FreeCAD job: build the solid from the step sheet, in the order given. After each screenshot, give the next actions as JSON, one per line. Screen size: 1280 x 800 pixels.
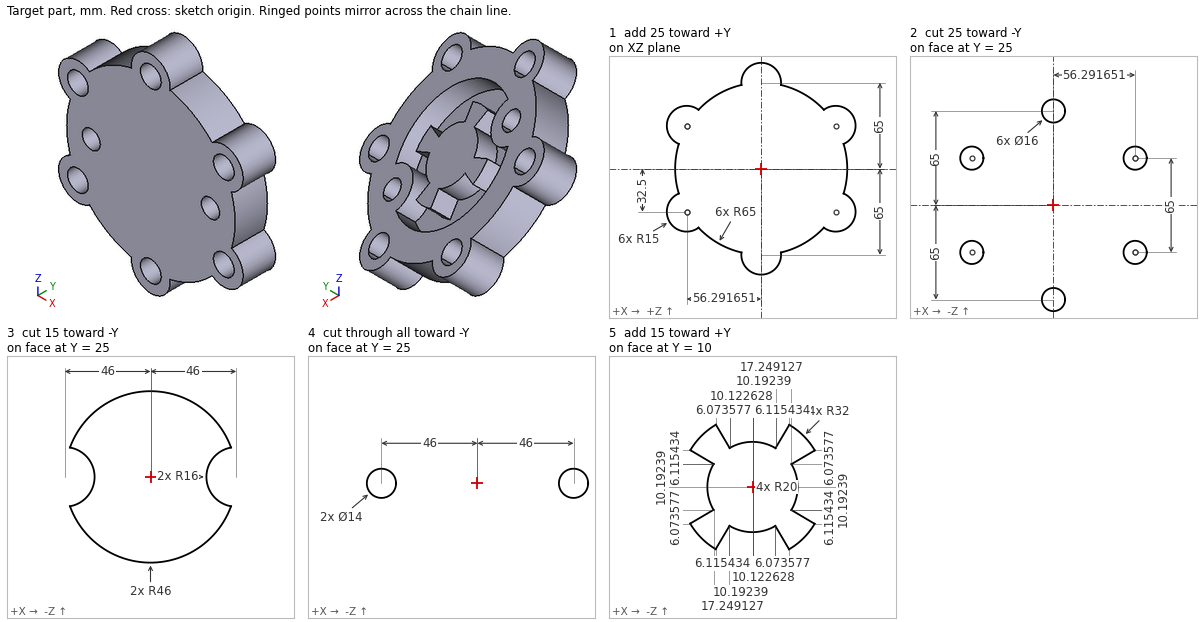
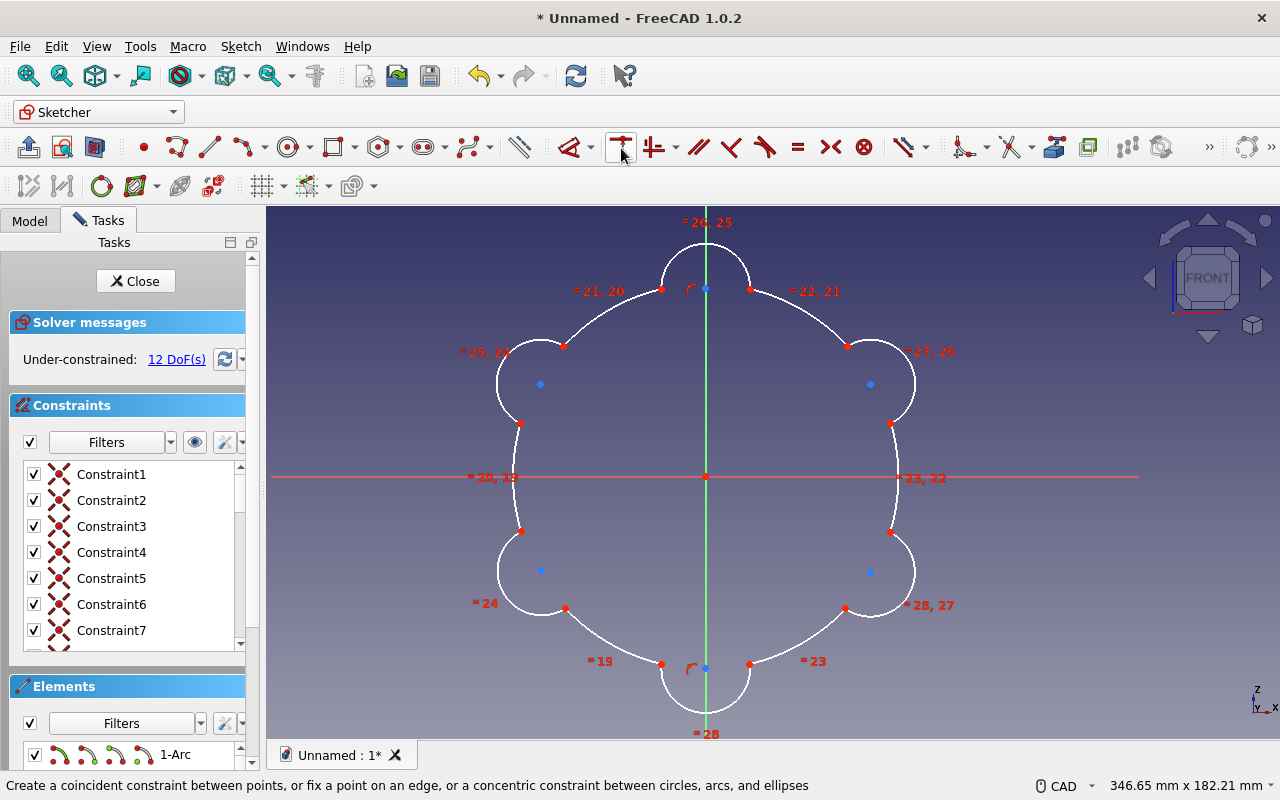
{"action": "left_click", "coordinate": [542, 571]}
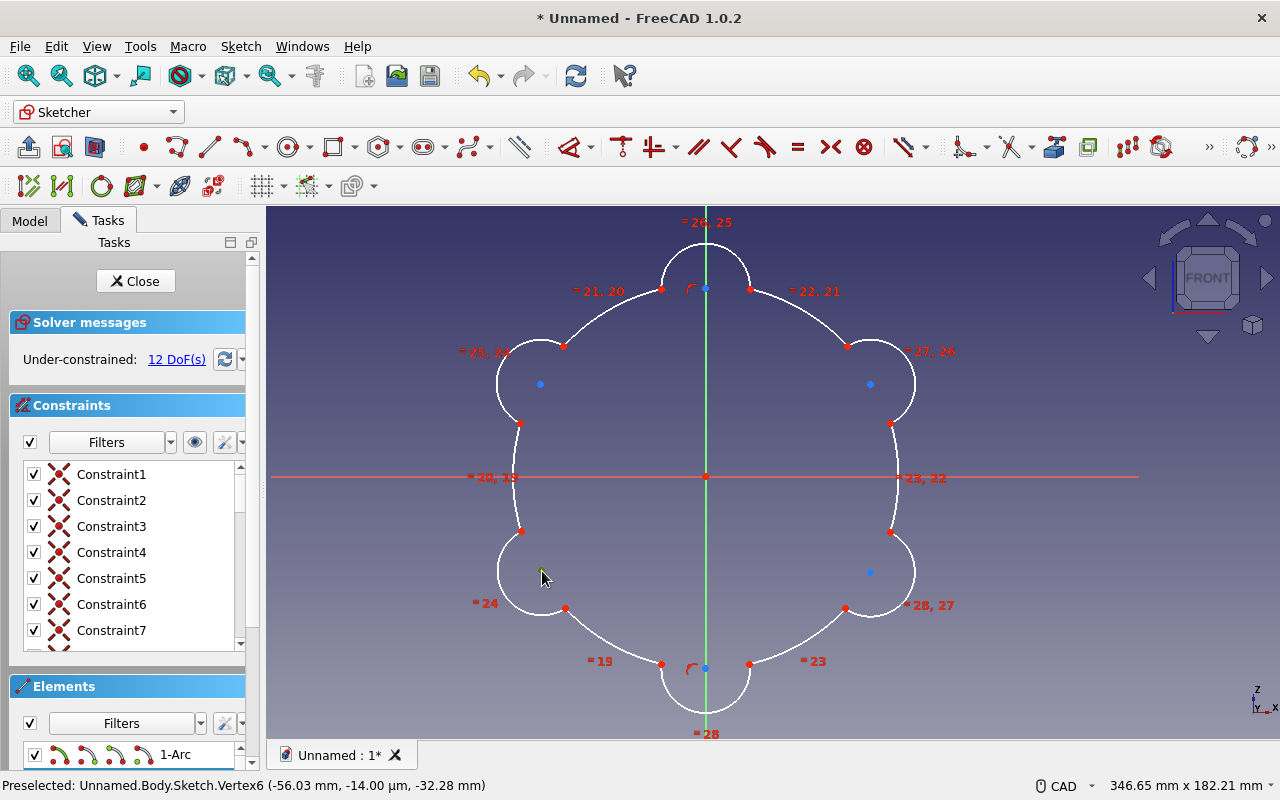
{"action": "left_click", "coordinate": [541, 384]}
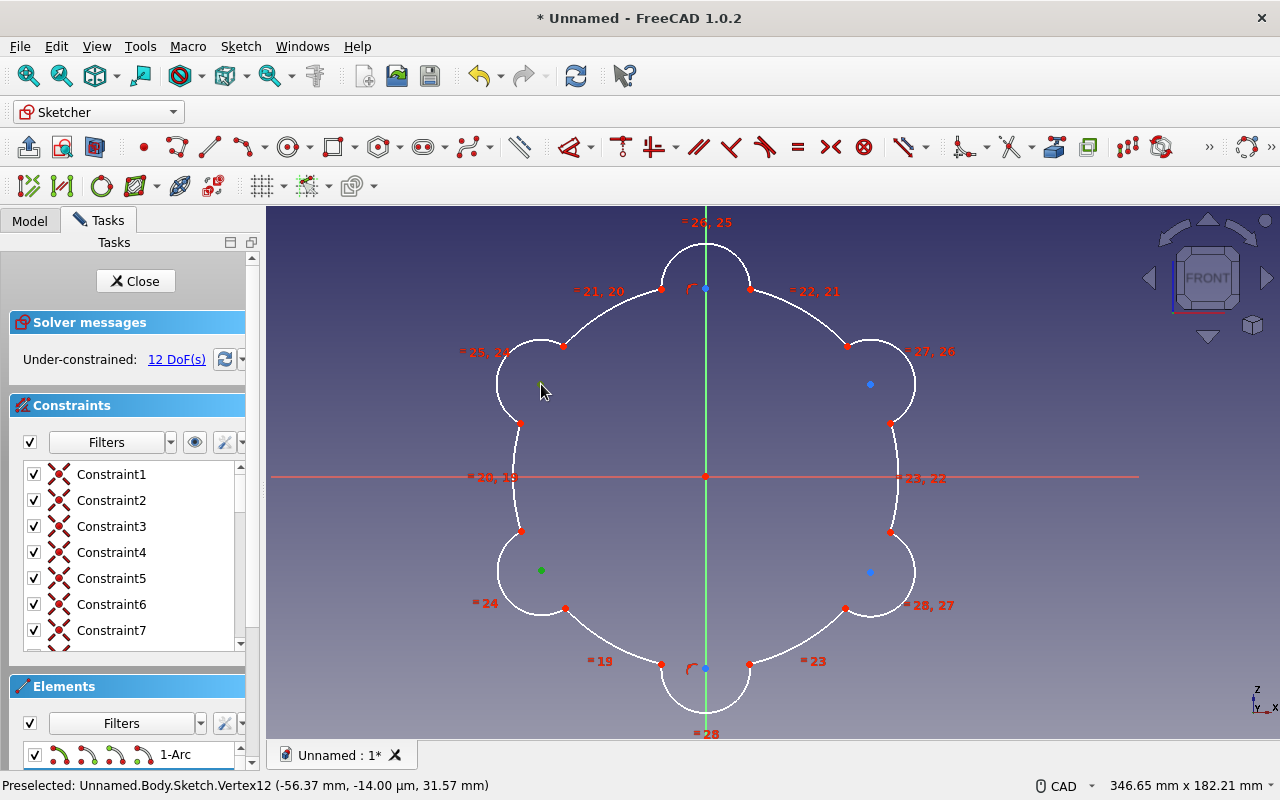
{"action": "left_click", "coordinate": [353, 477]}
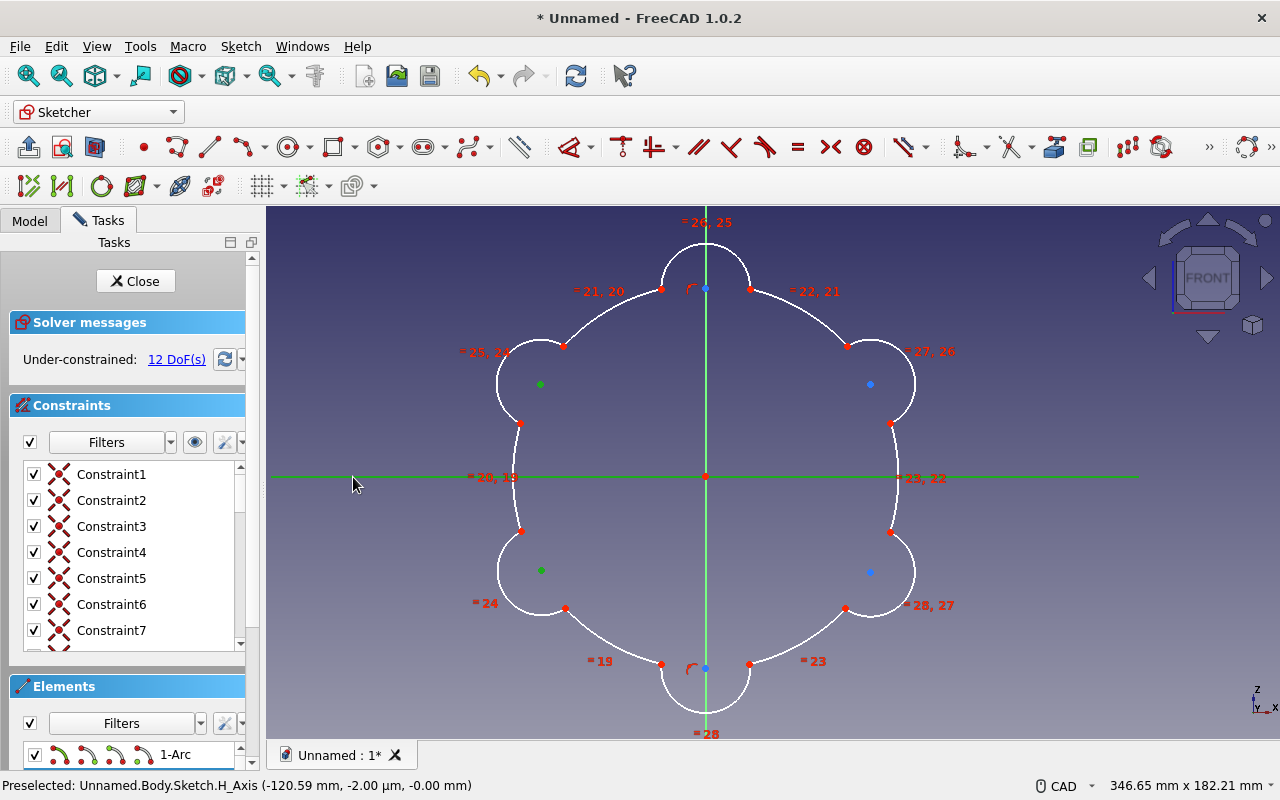
{"action": "left_click", "coordinate": [831, 148]}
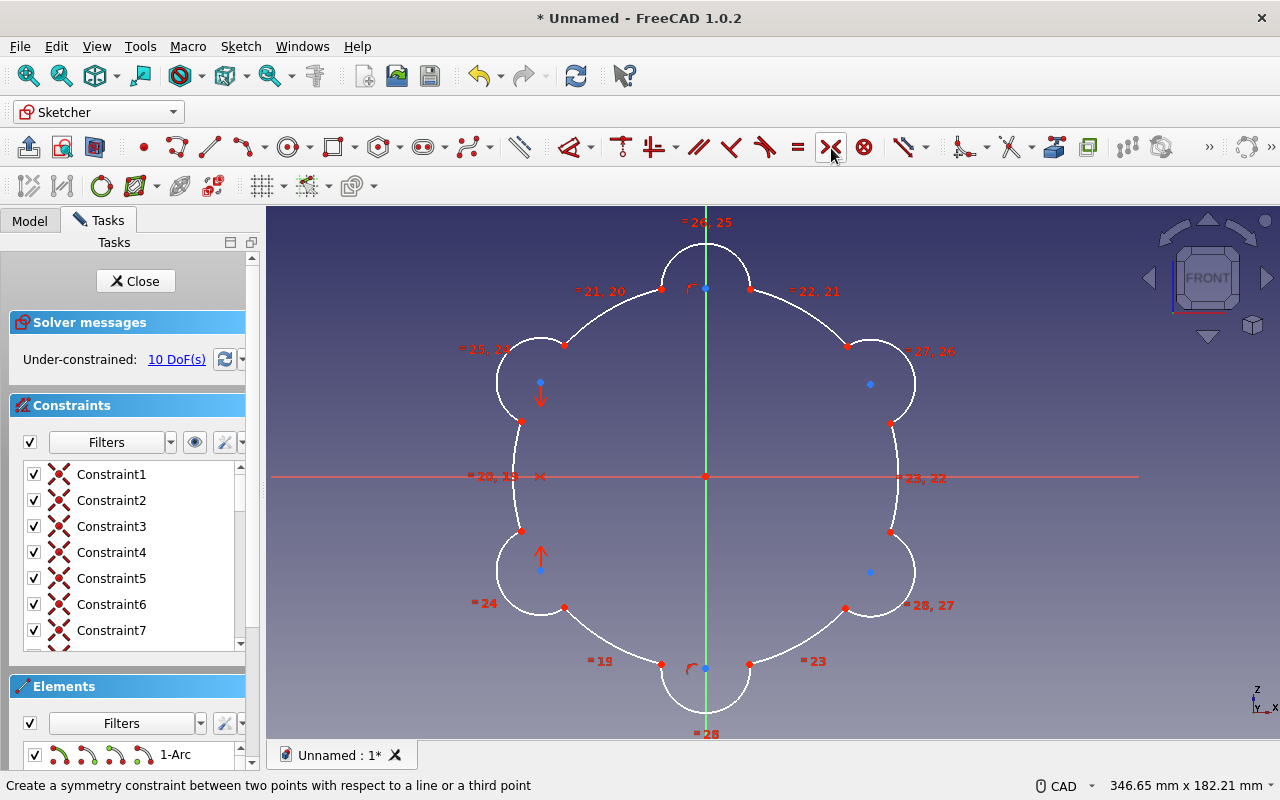
{"action": "left_click", "coordinate": [541, 382]}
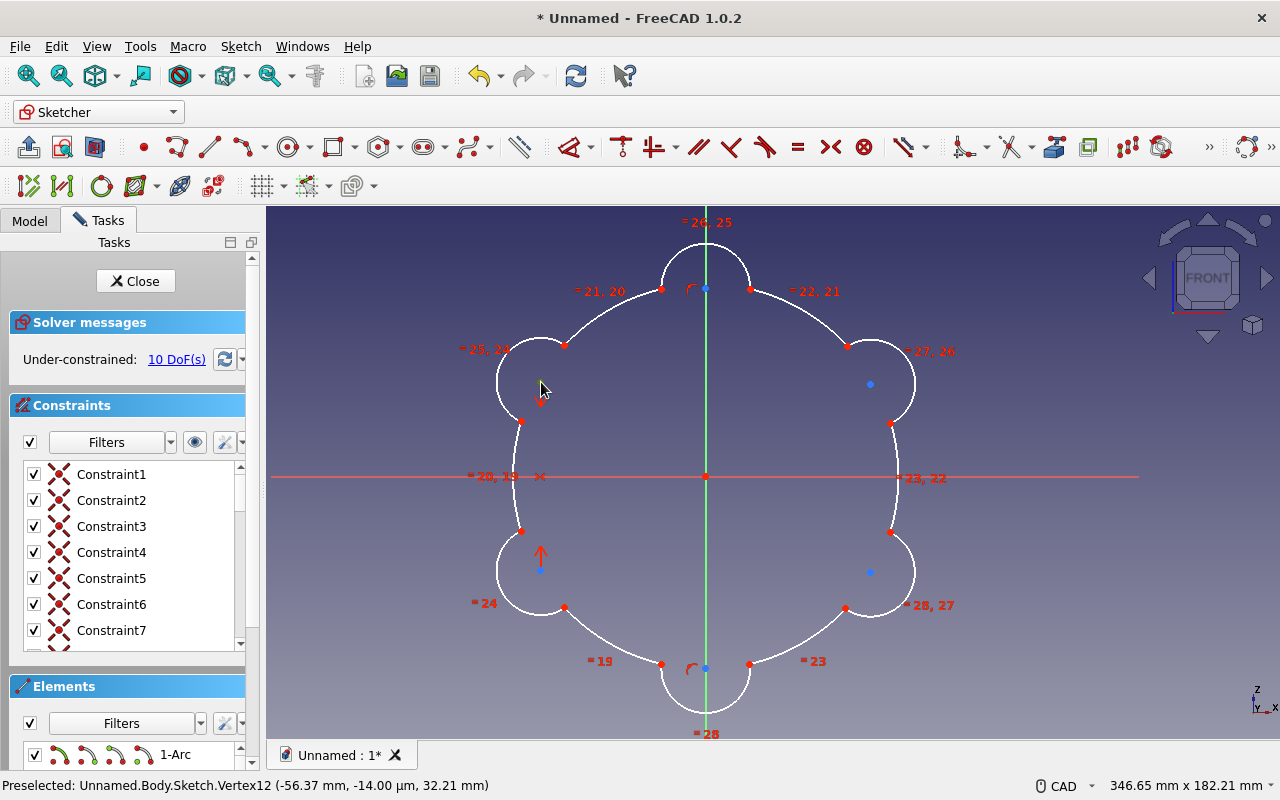
{"action": "left_click", "coordinate": [871, 384]}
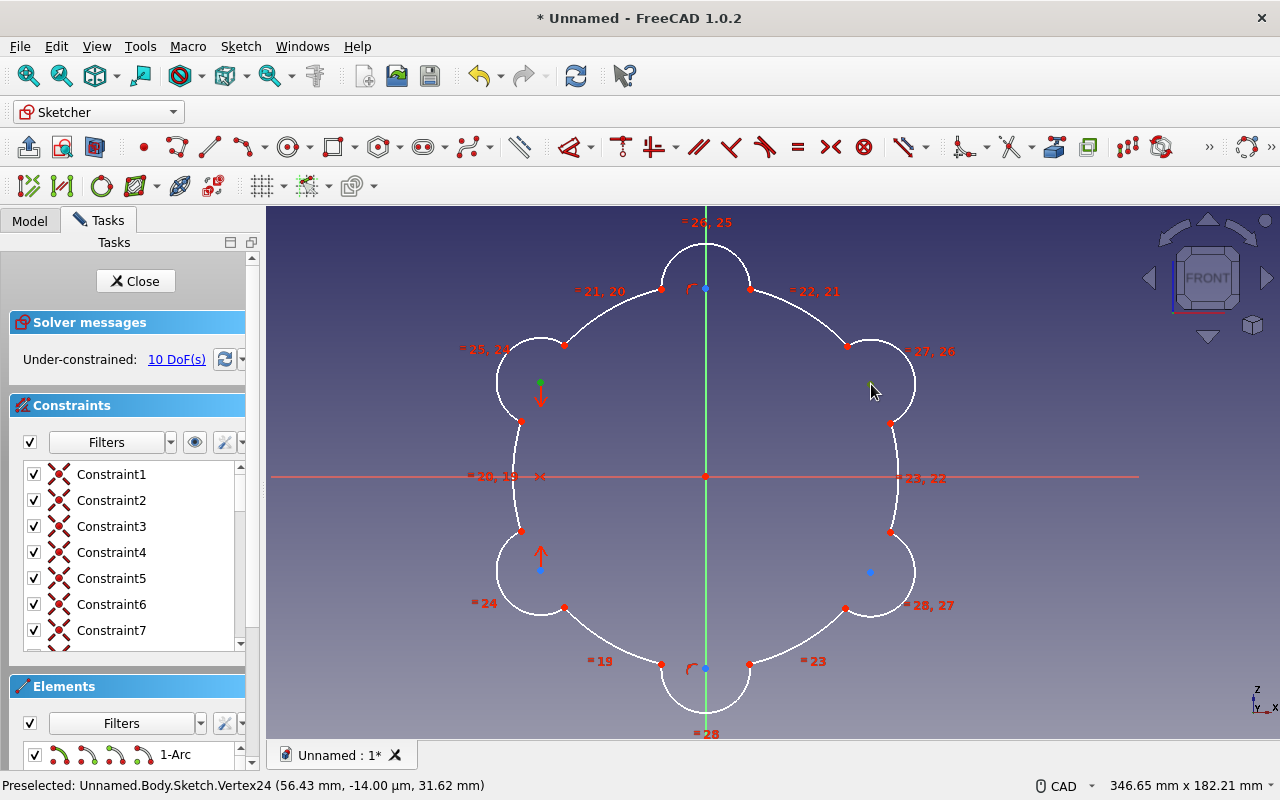
{"action": "left_click", "coordinate": [706, 677]}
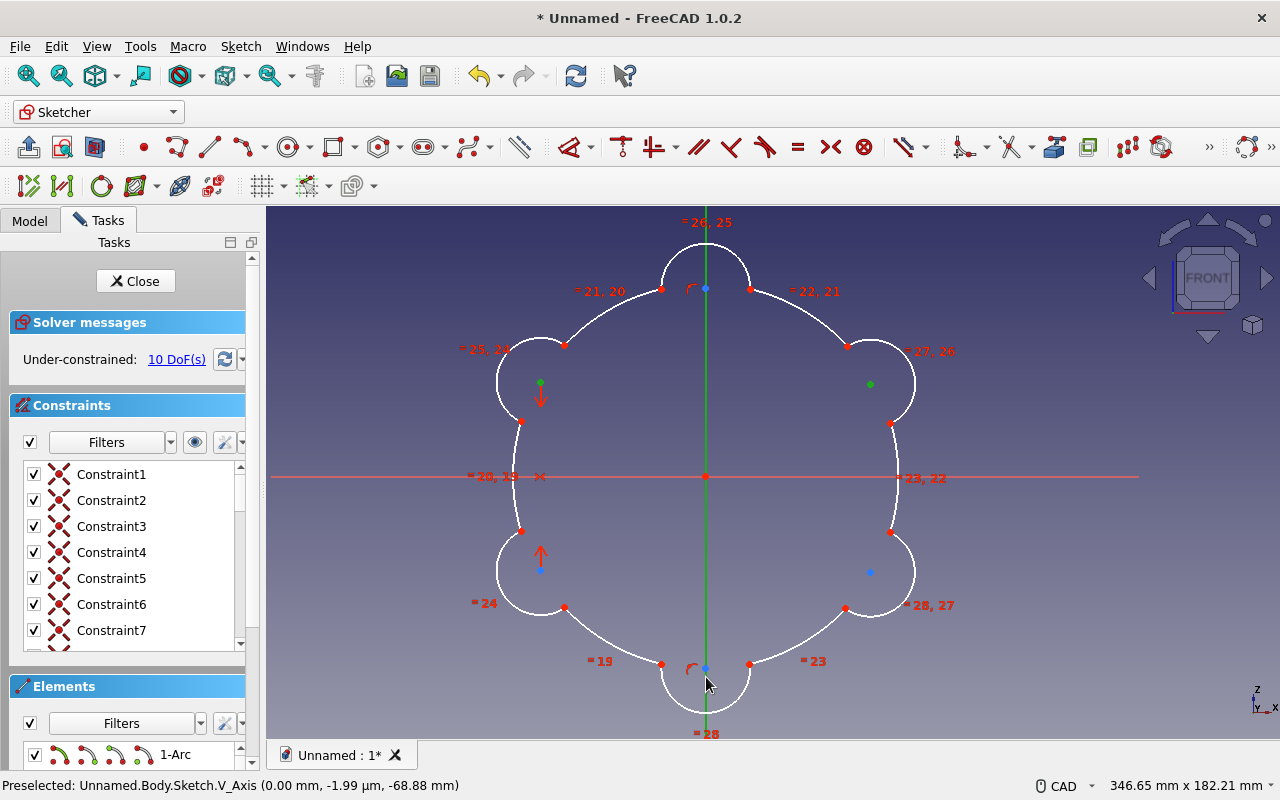
{"action": "left_click", "coordinate": [831, 148]}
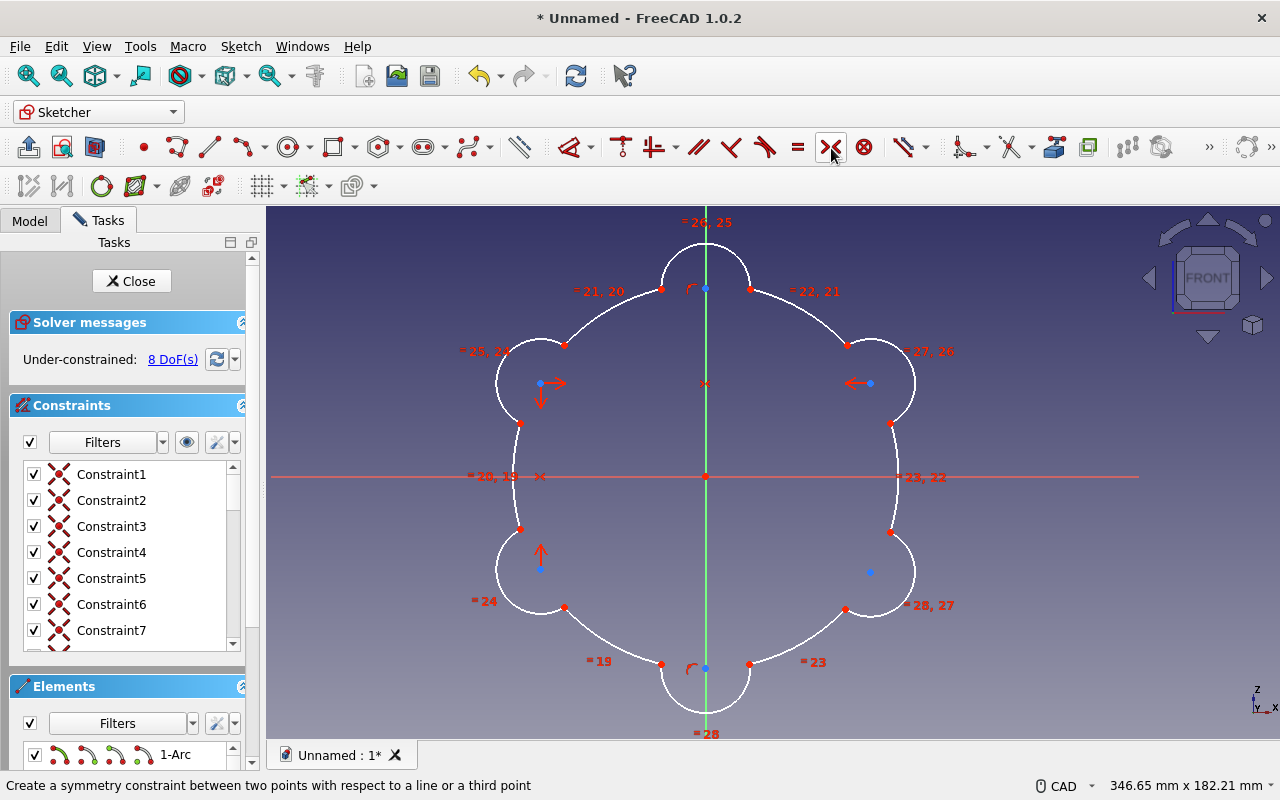
{"action": "left_click", "coordinate": [541, 570]}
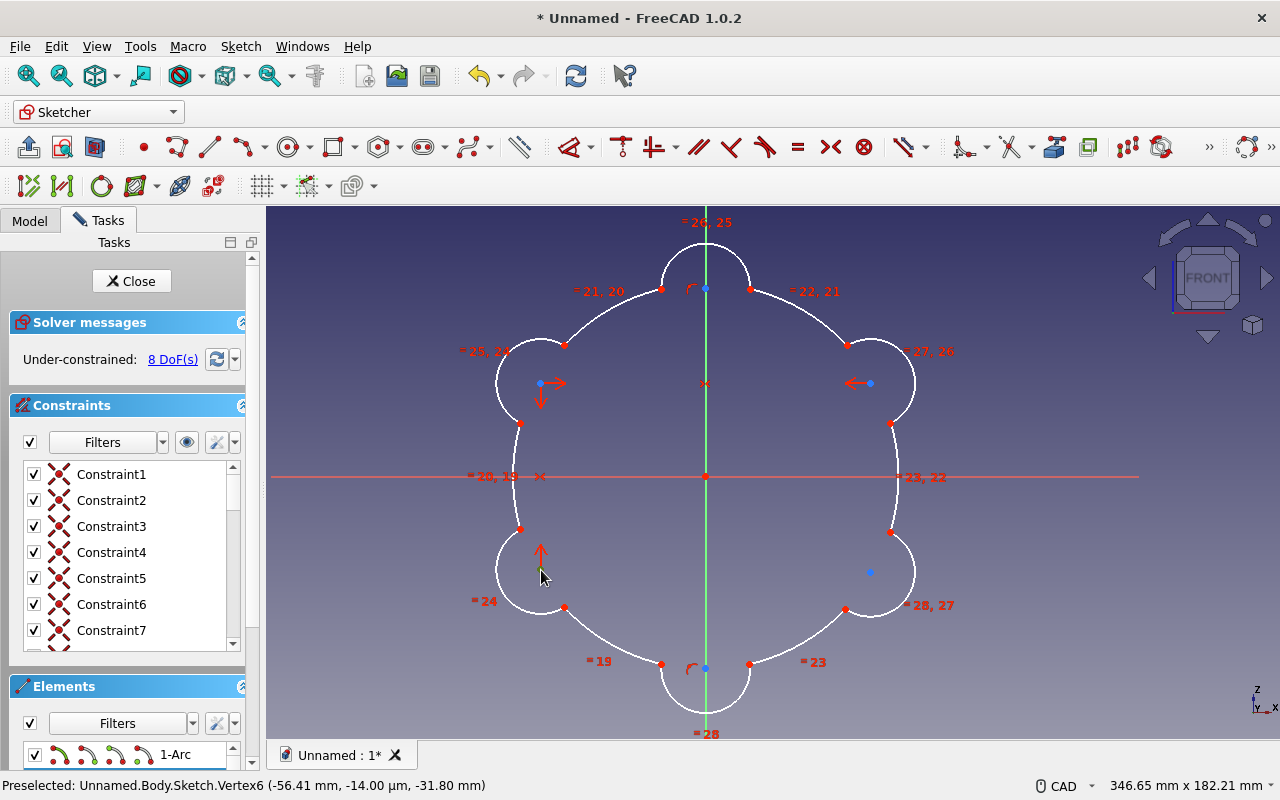
{"action": "left_click", "coordinate": [870, 572]}